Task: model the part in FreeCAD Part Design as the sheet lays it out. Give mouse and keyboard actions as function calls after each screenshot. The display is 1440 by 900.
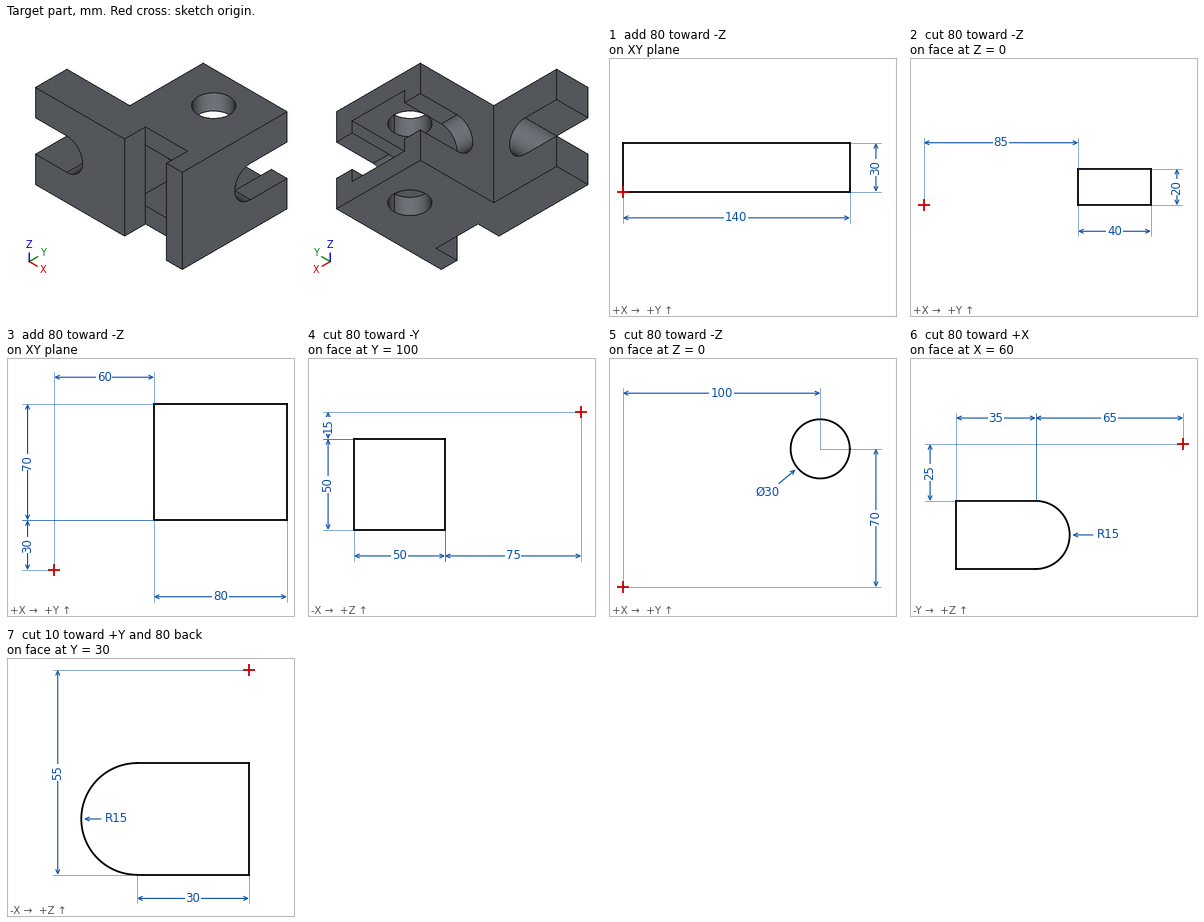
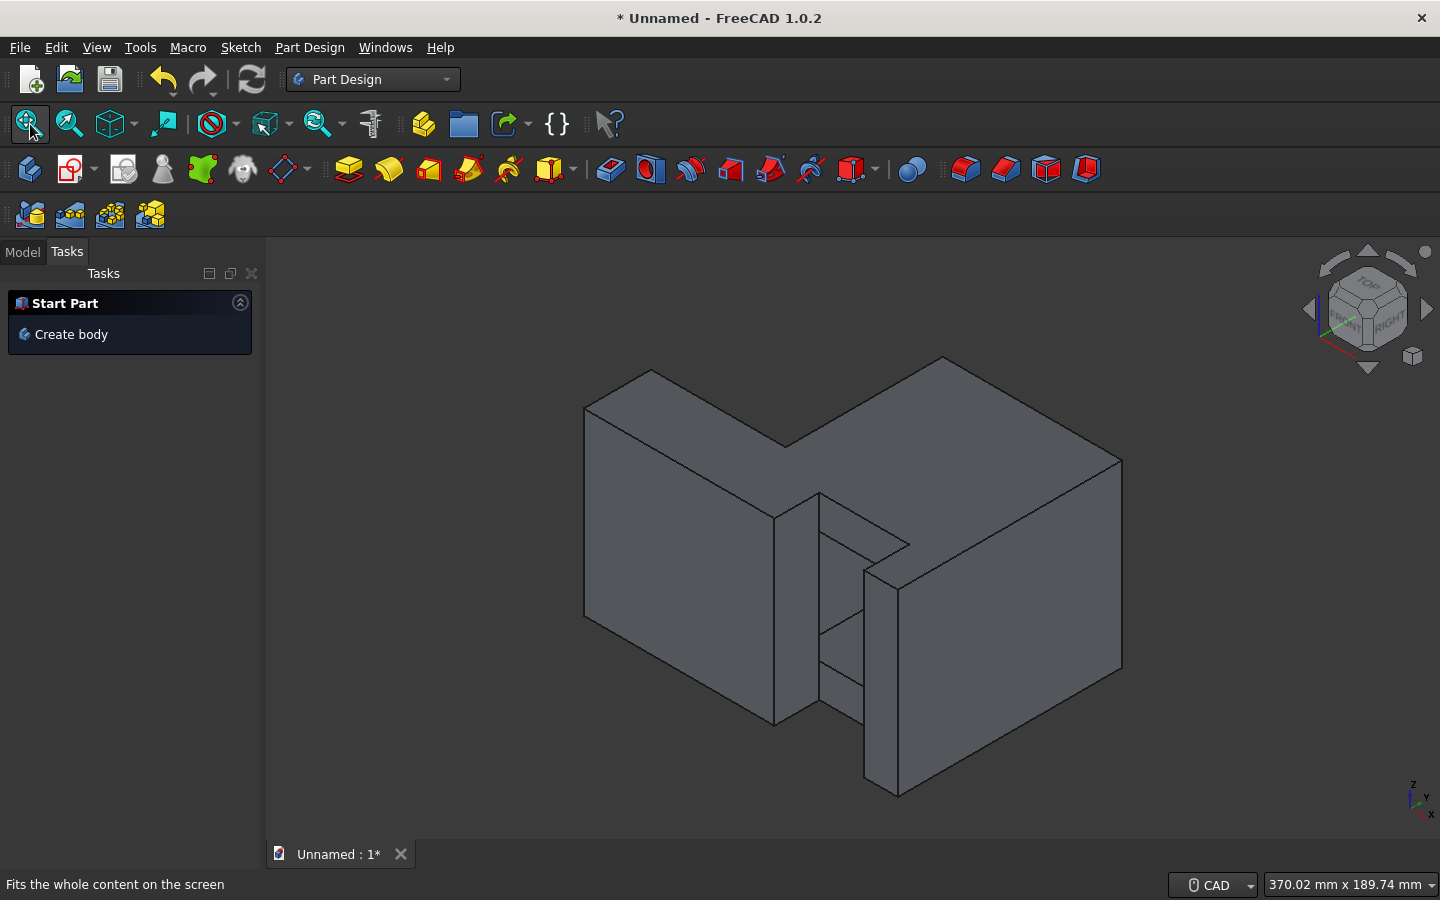
click(975, 467)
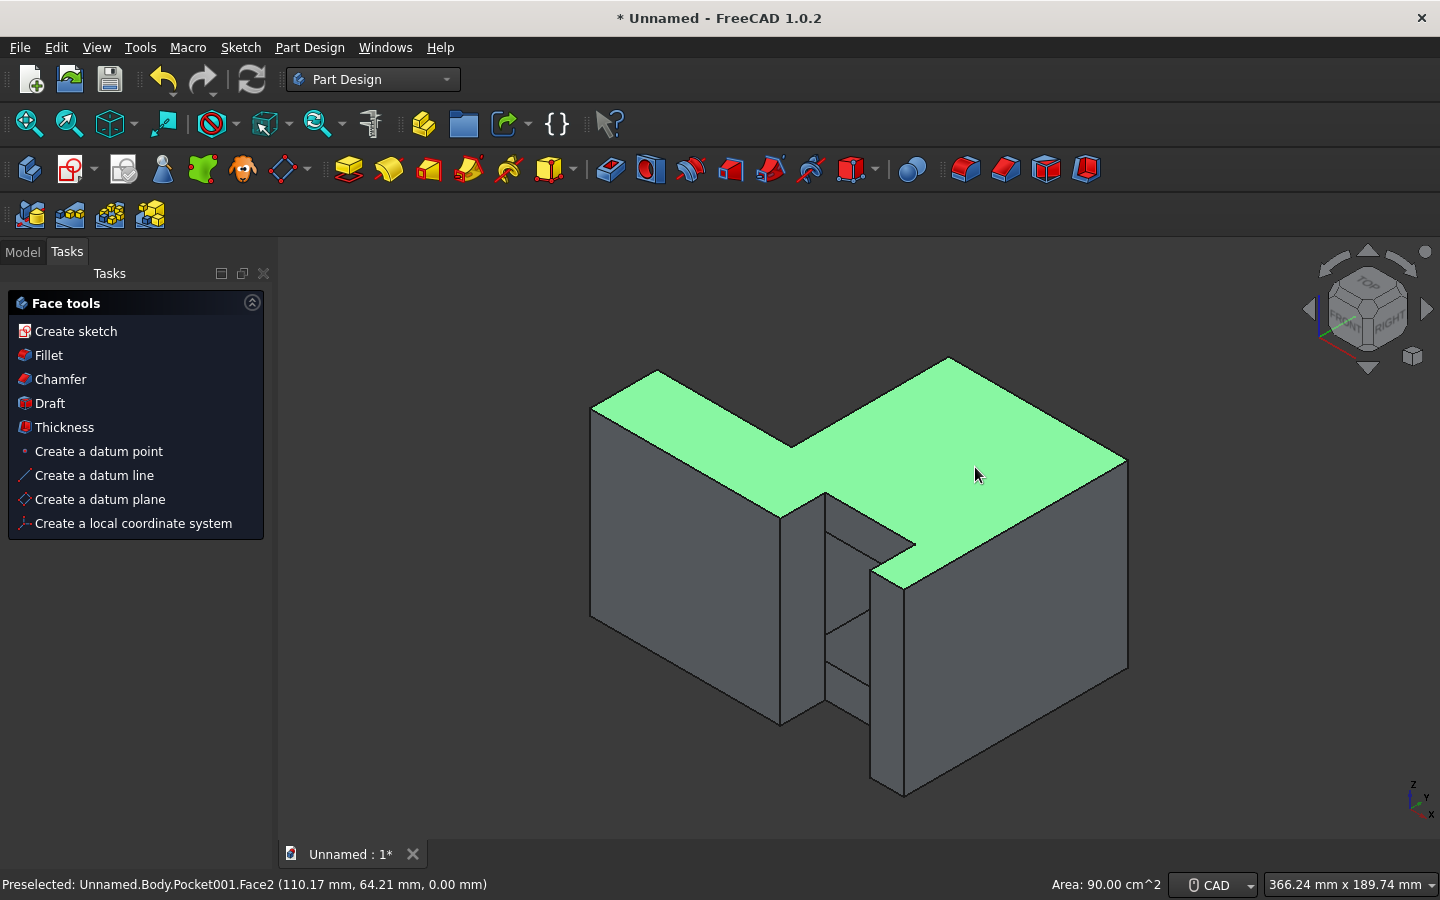
click(70, 170)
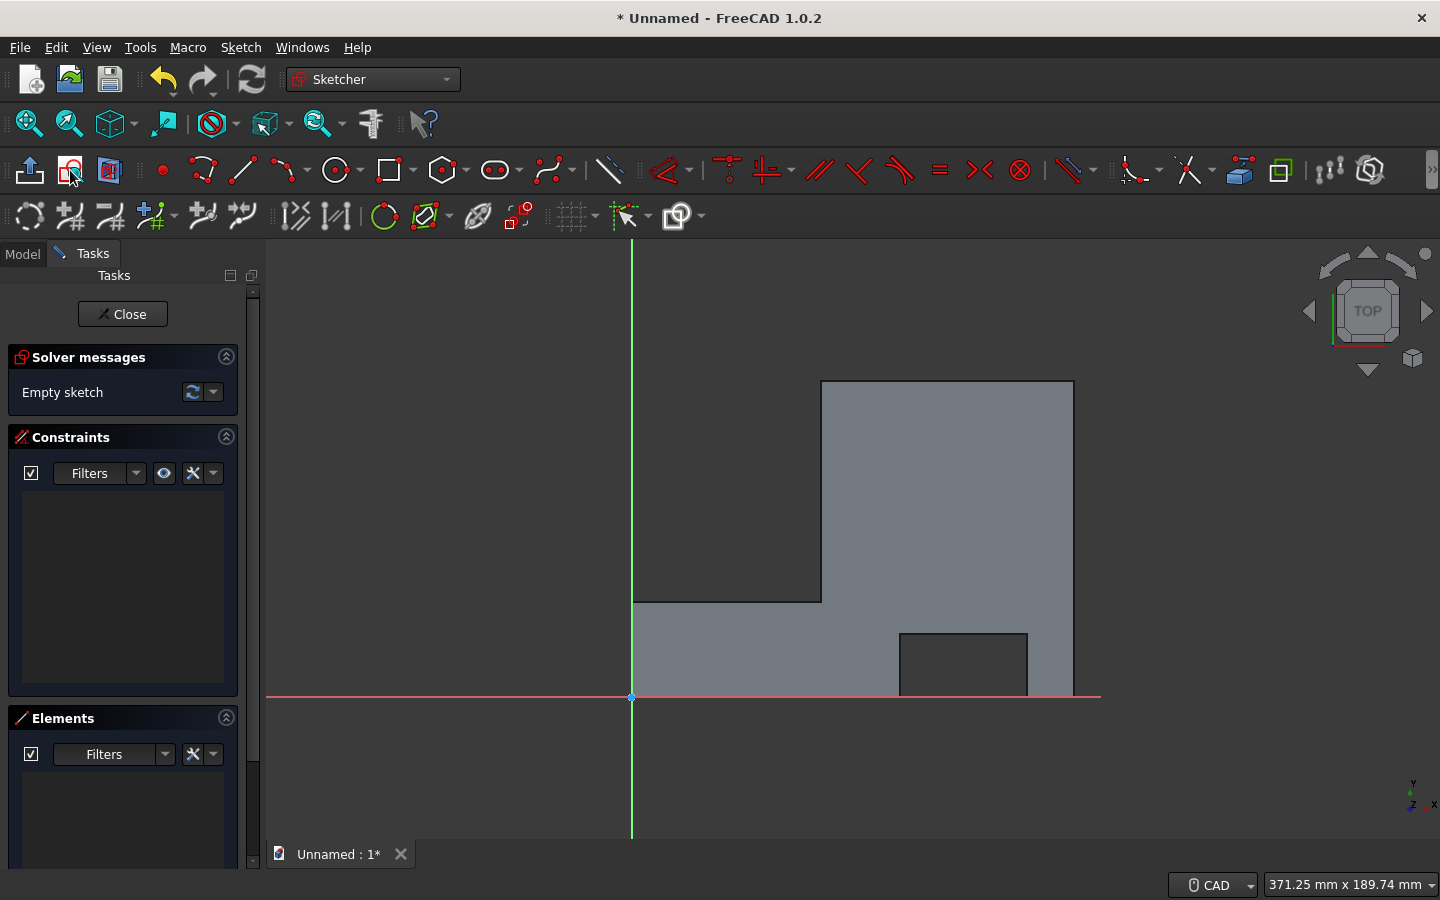
scroll(1001, 455, up, 7)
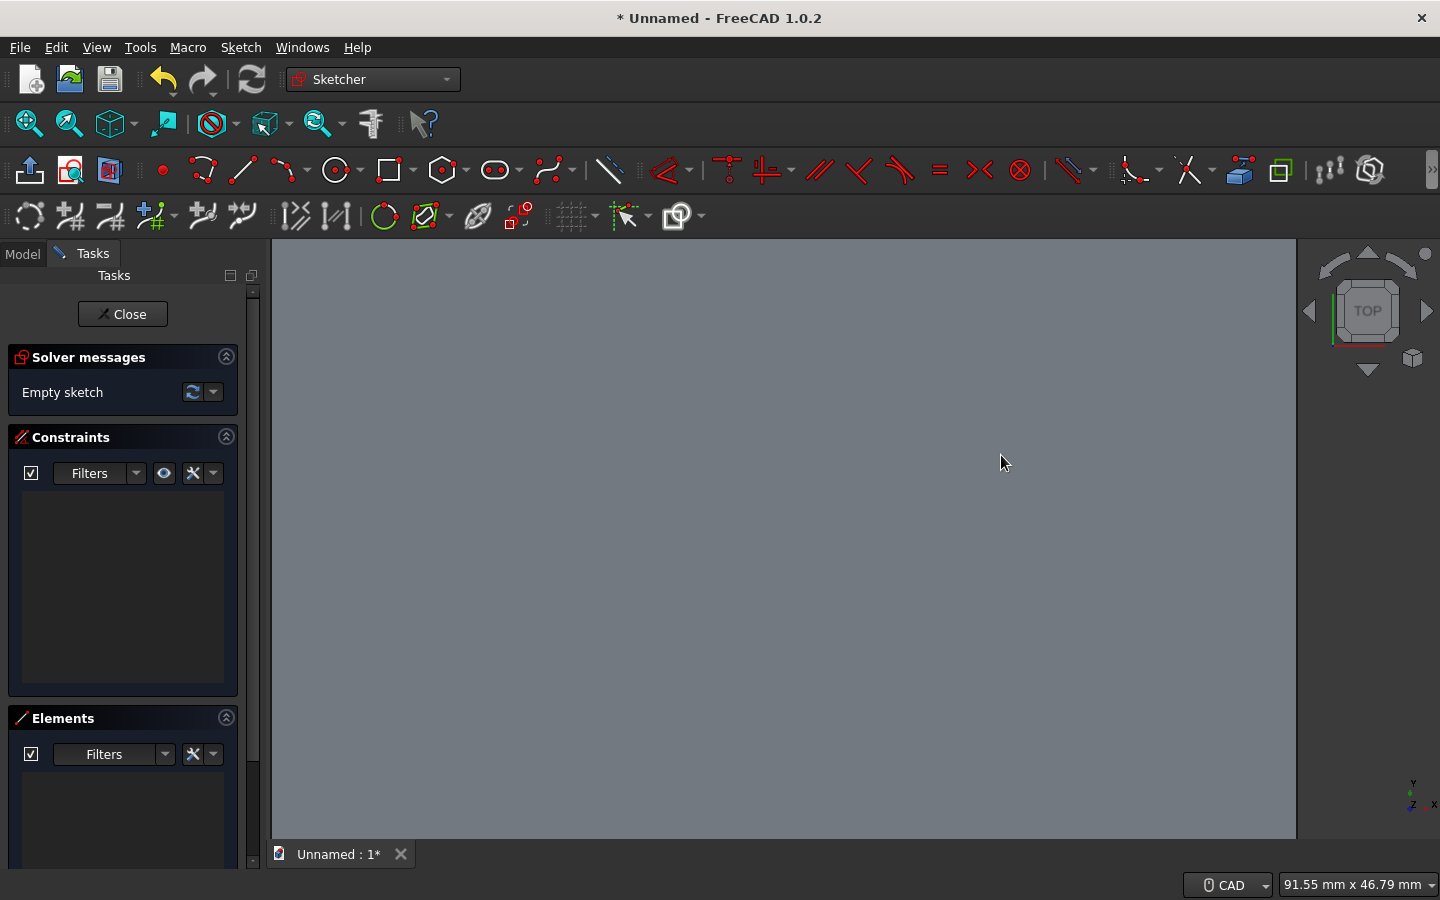
key(g)
key(c)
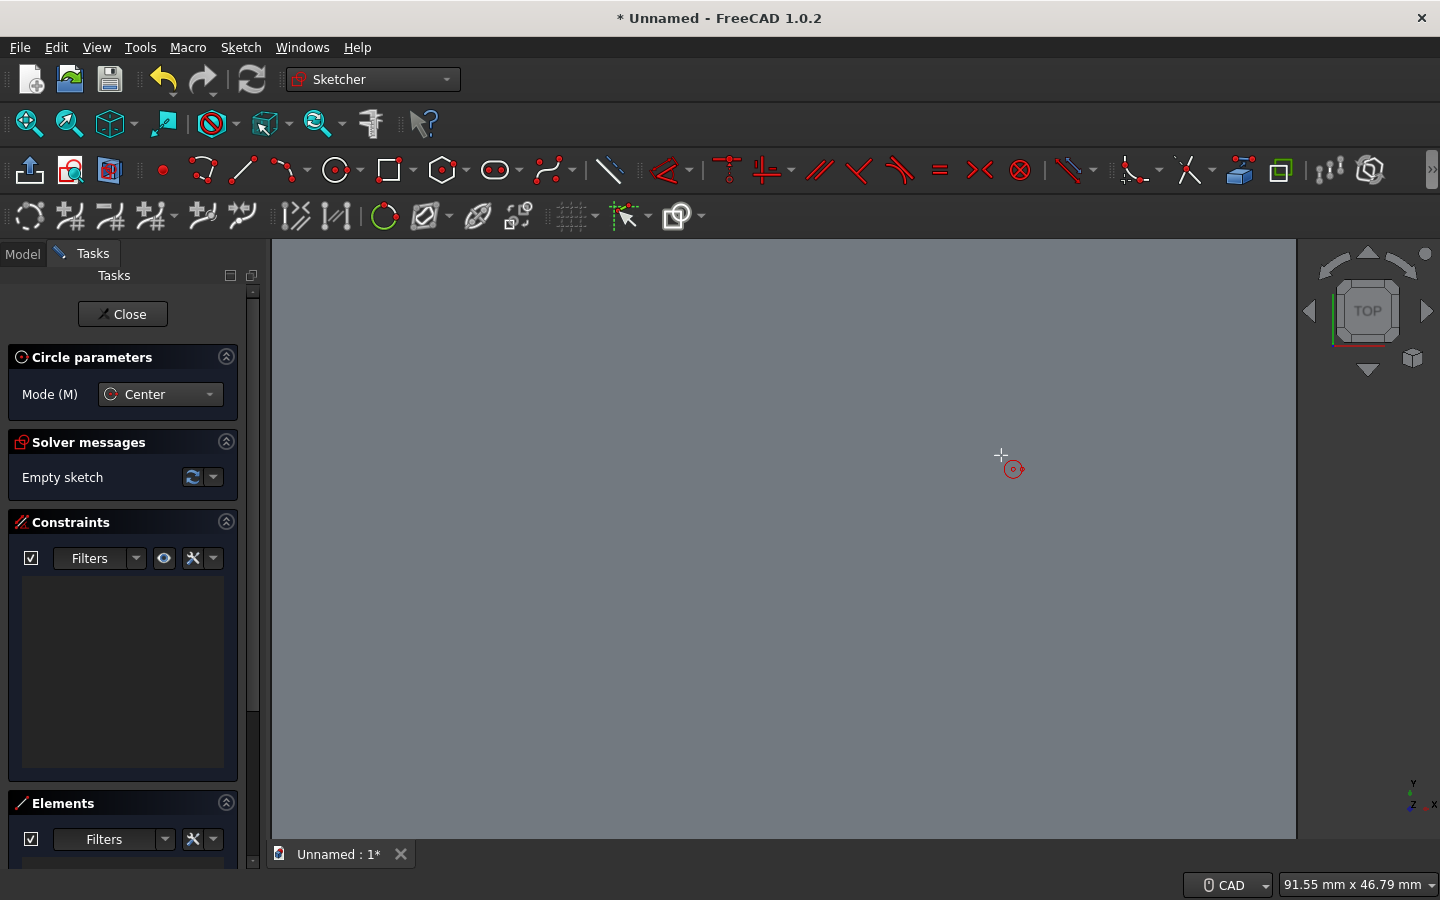
click(784, 538)
click(920, 402)
key(Escape)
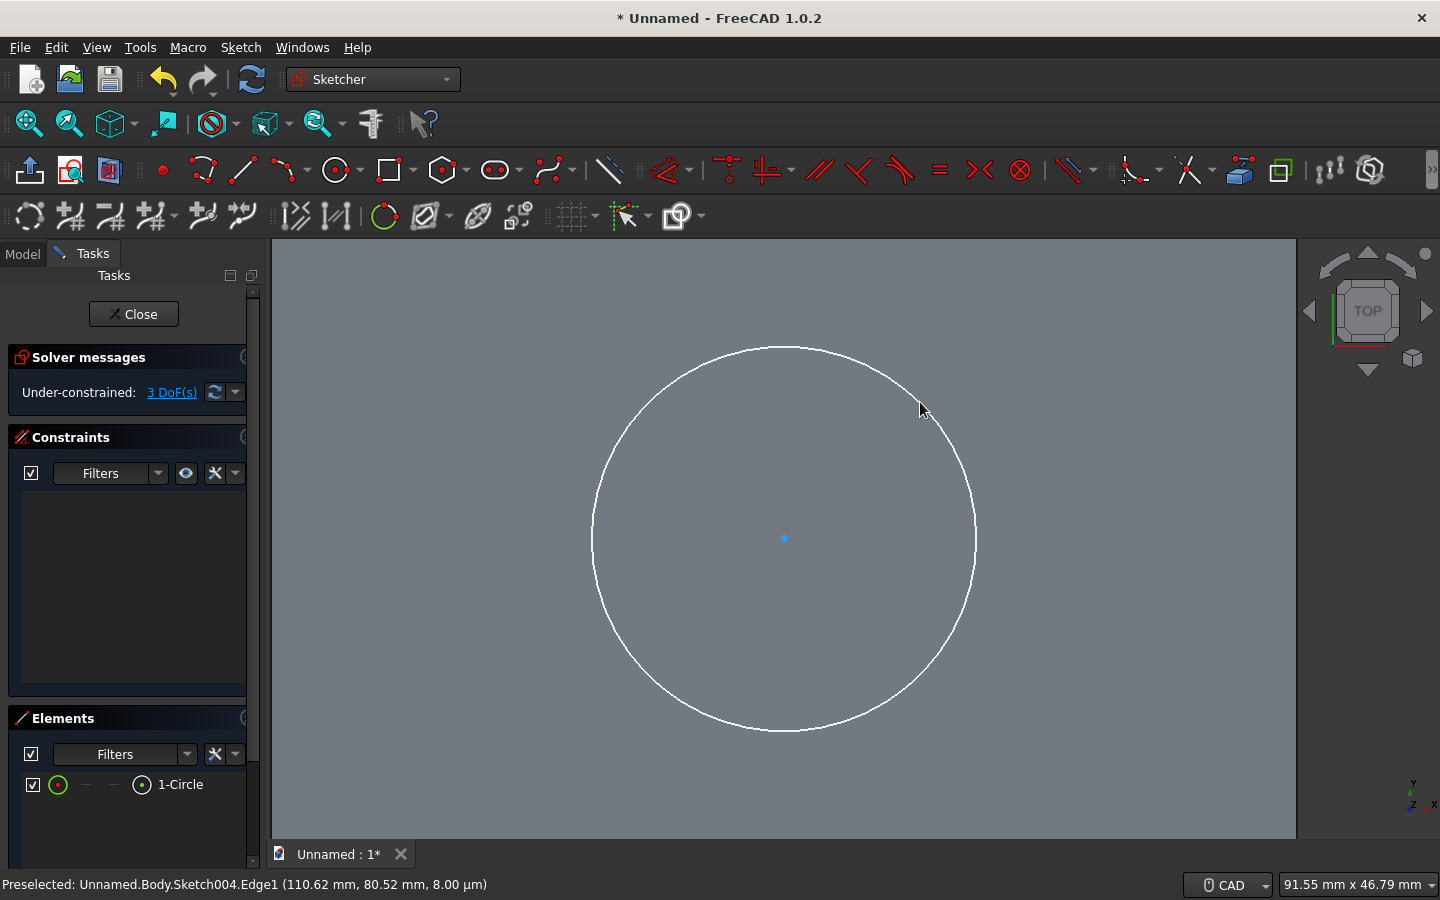
key(d)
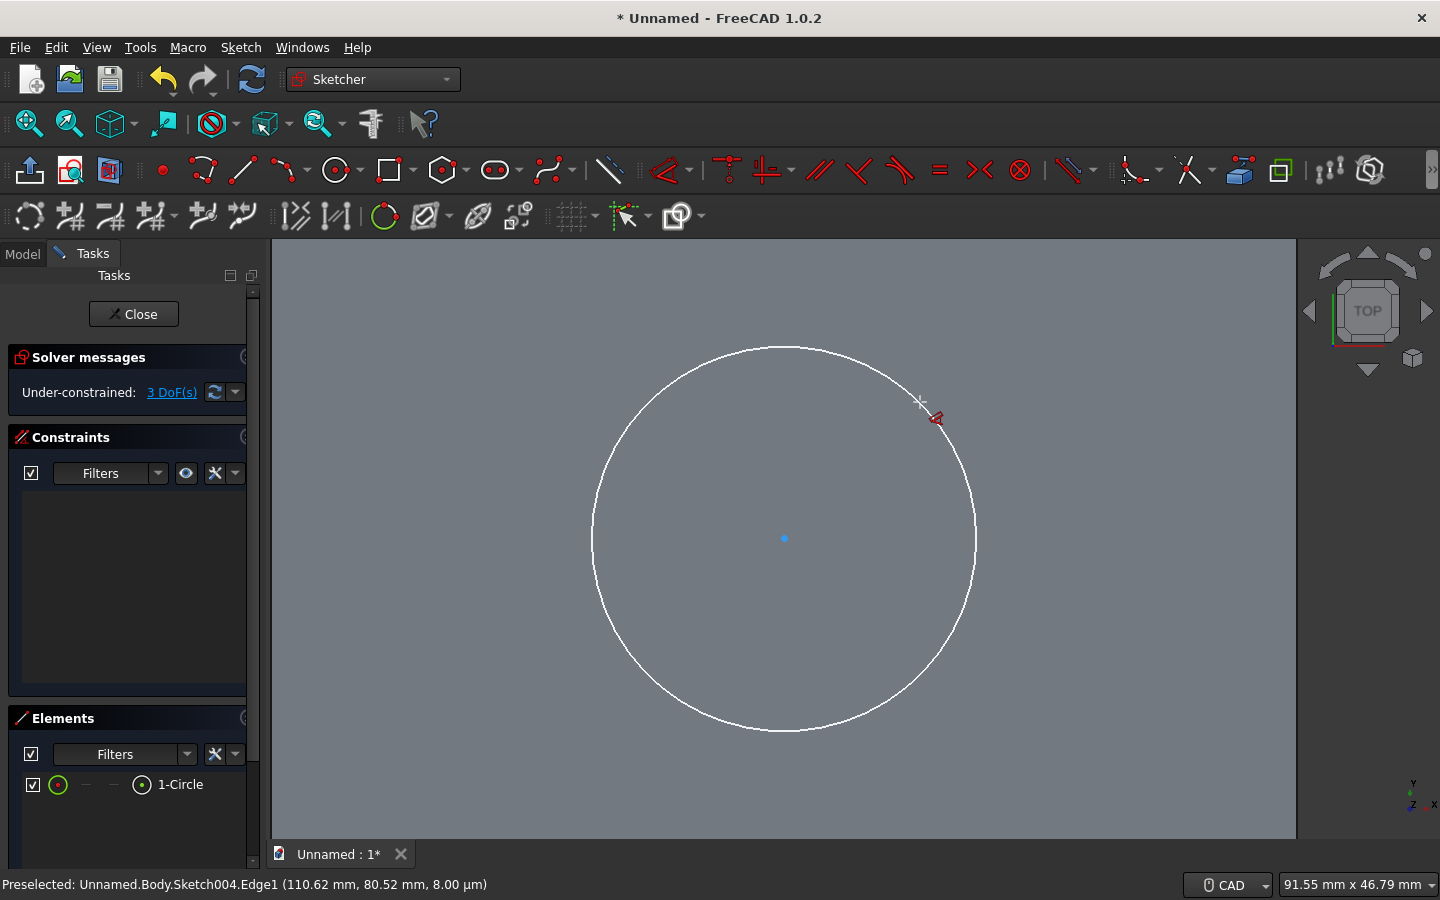
click(920, 403)
click(943, 380)